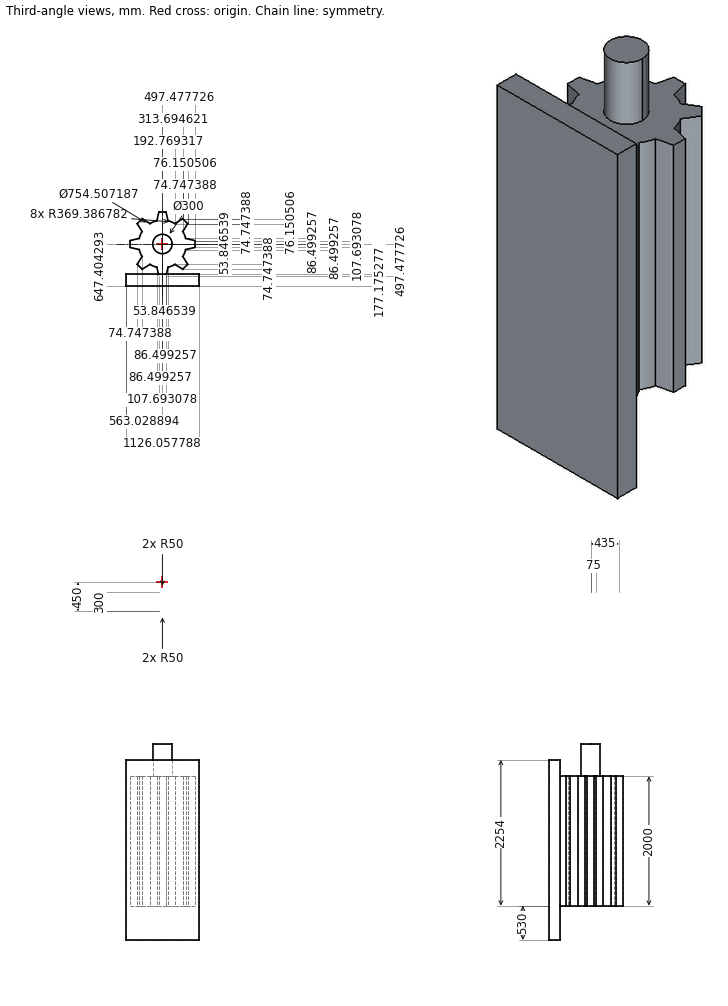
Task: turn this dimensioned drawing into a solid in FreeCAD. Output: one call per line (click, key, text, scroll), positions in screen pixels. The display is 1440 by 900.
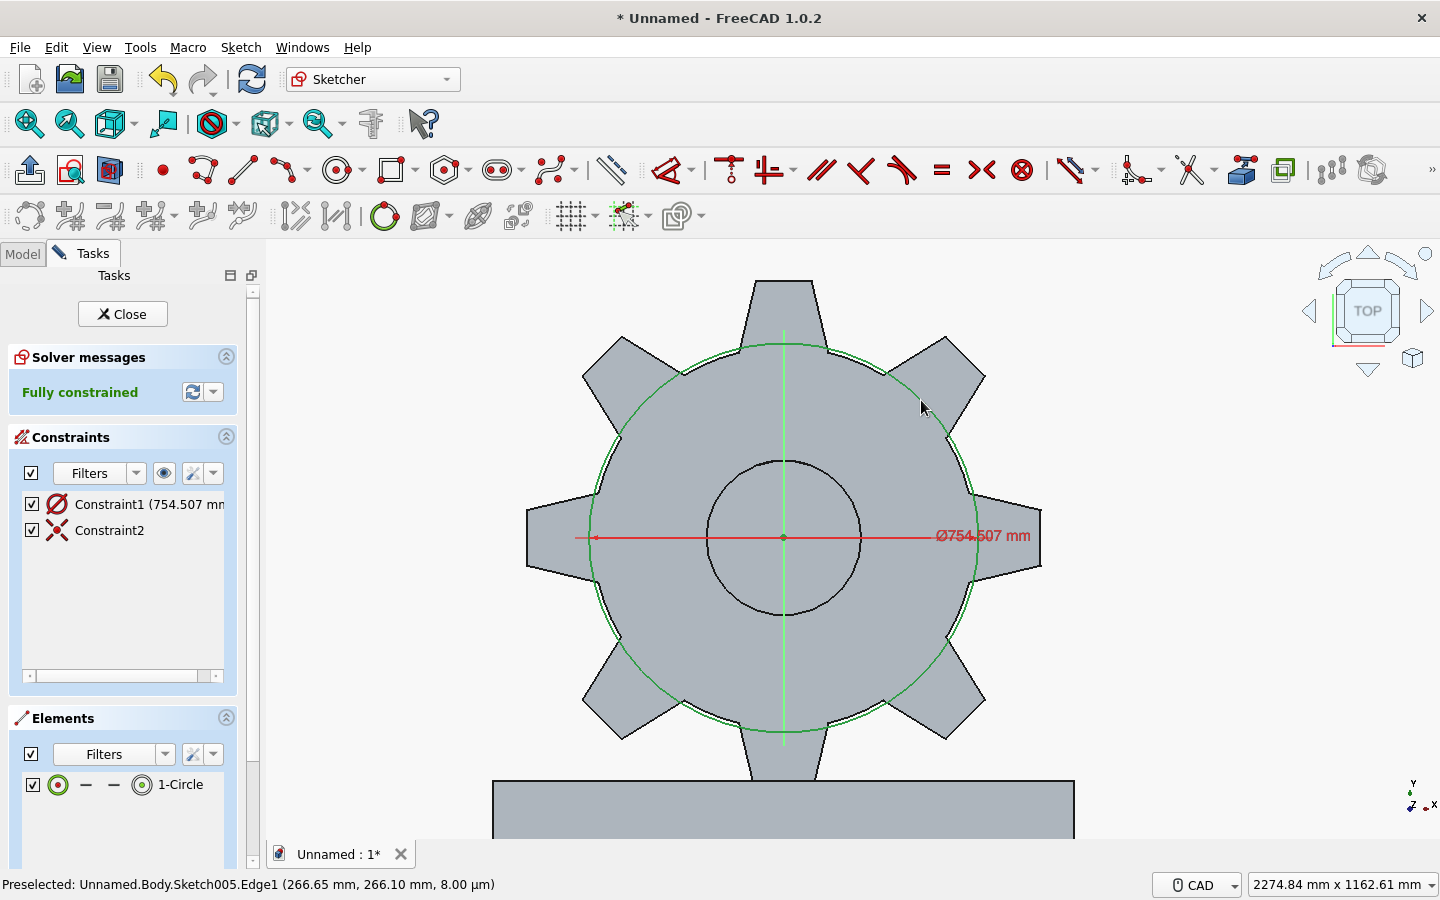
click(123, 314)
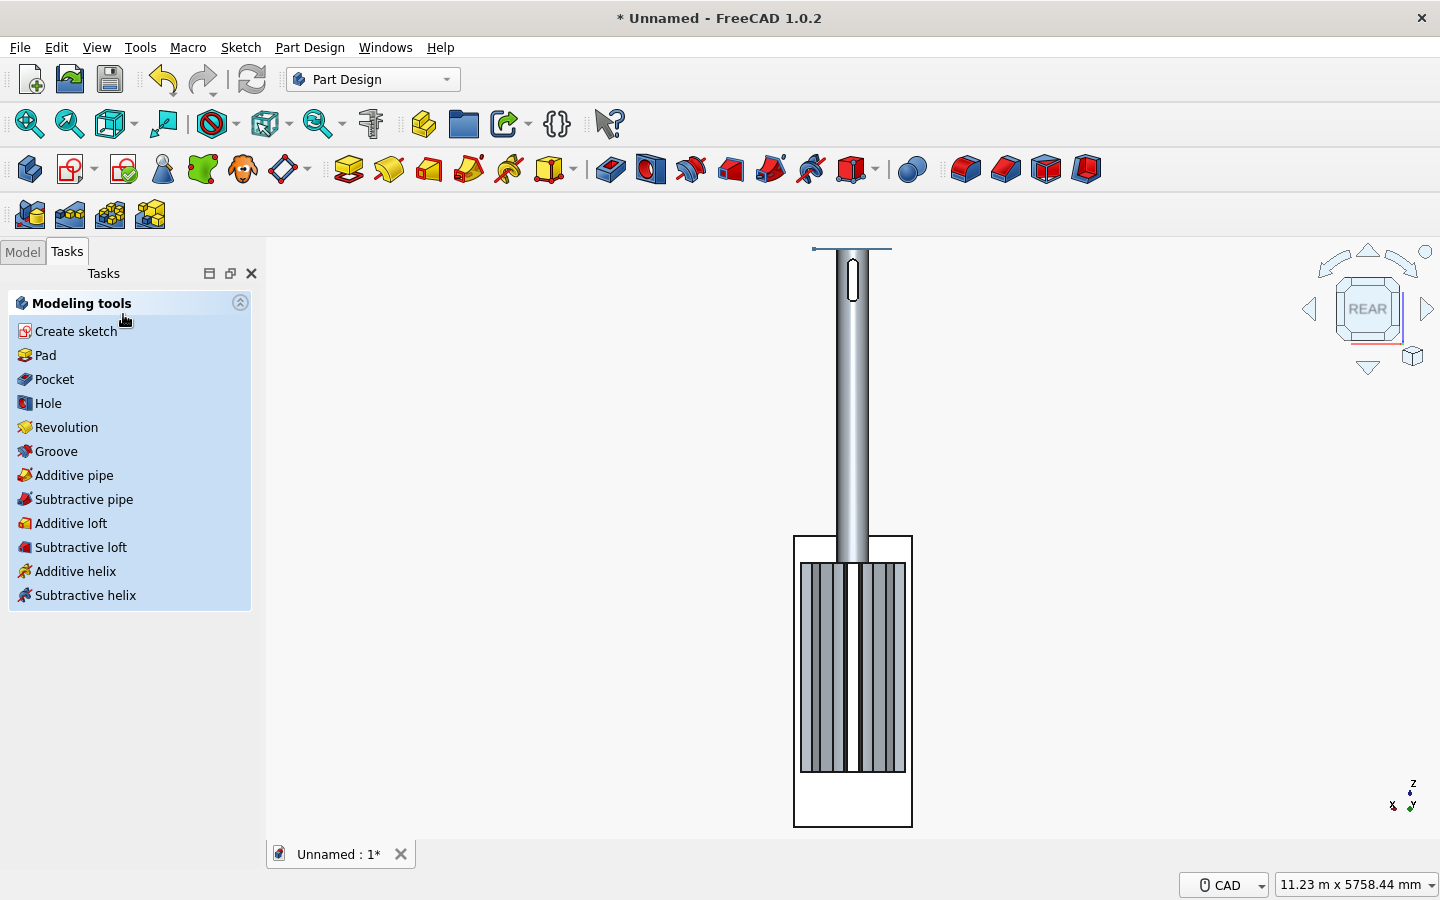
click(612, 170)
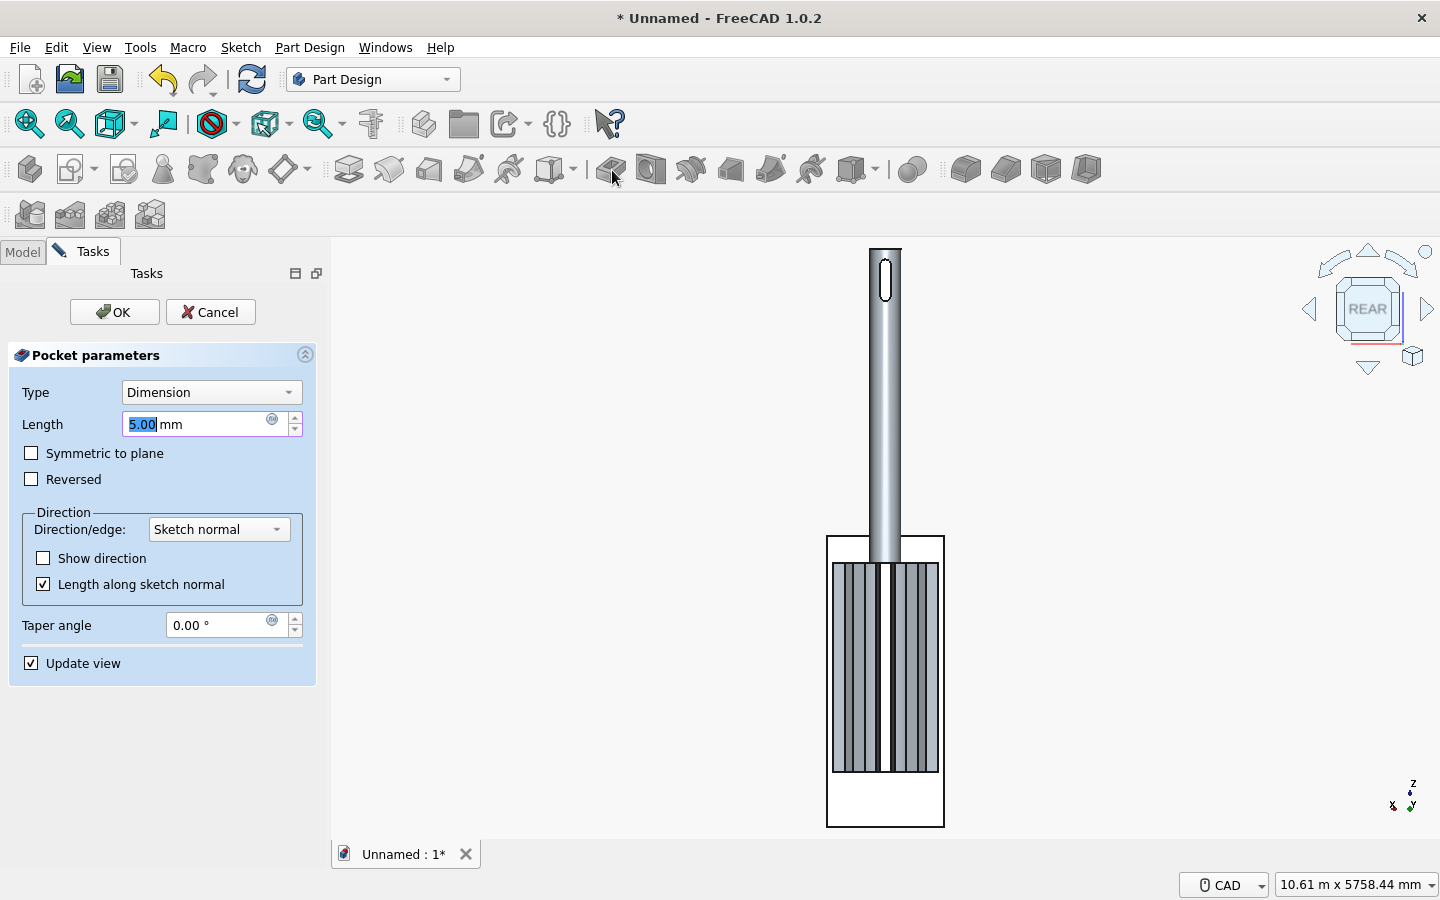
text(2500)
key(Tab)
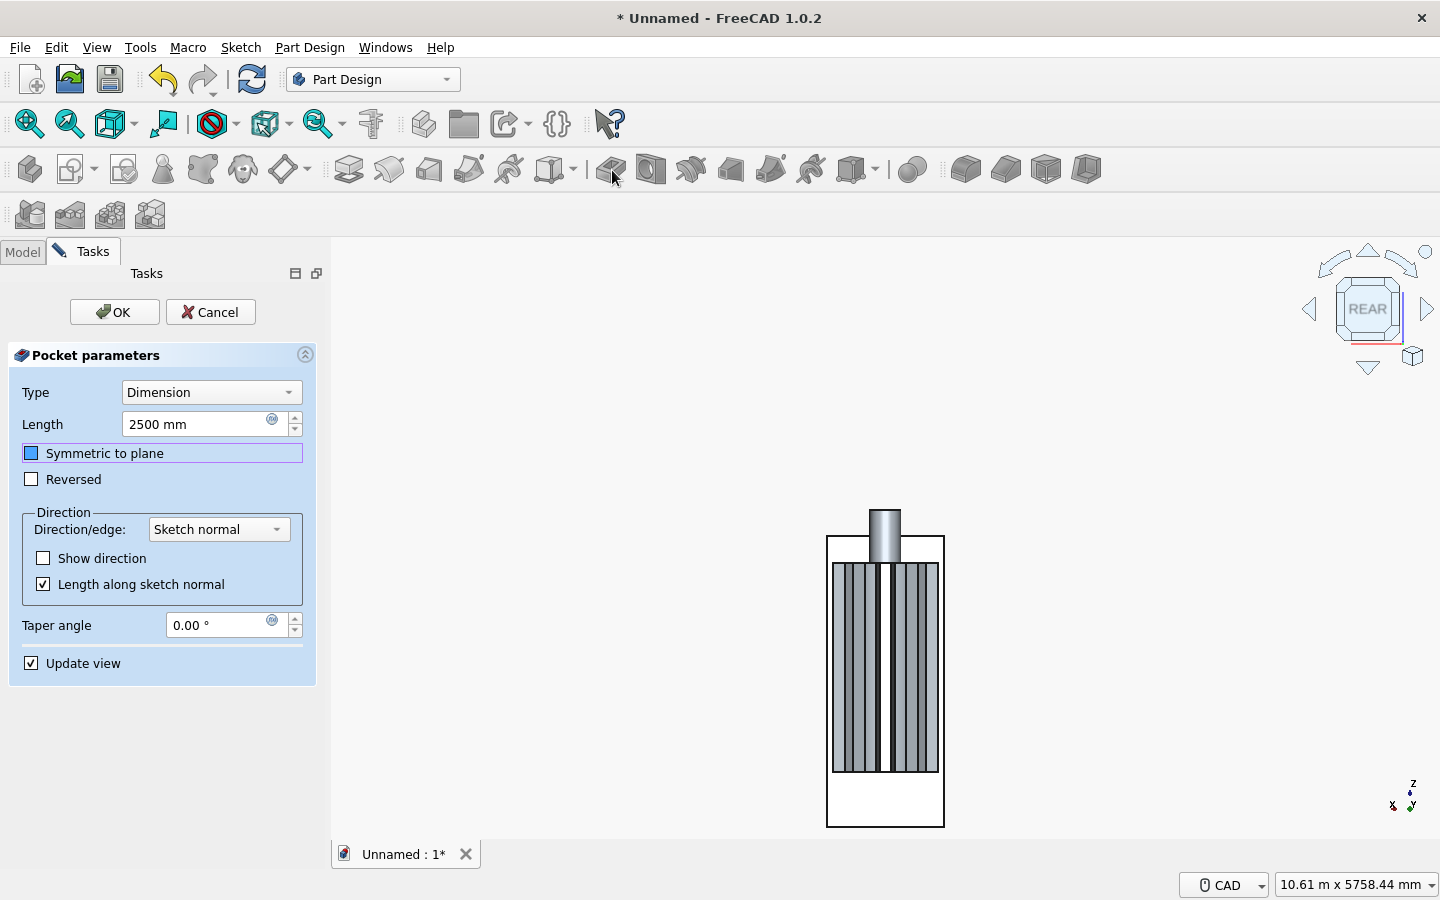
click(115, 312)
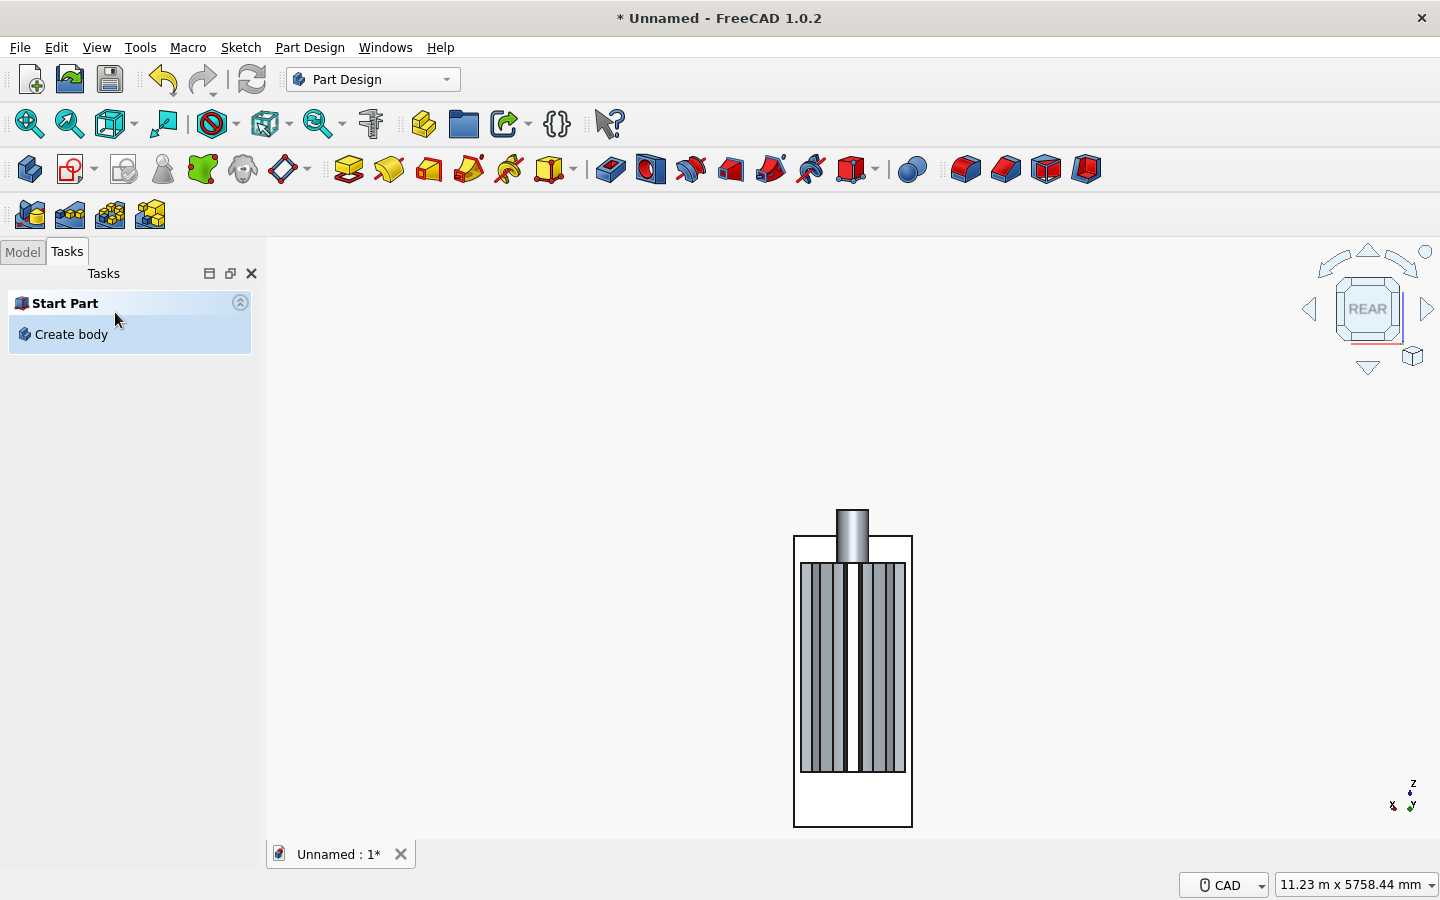
key(0)